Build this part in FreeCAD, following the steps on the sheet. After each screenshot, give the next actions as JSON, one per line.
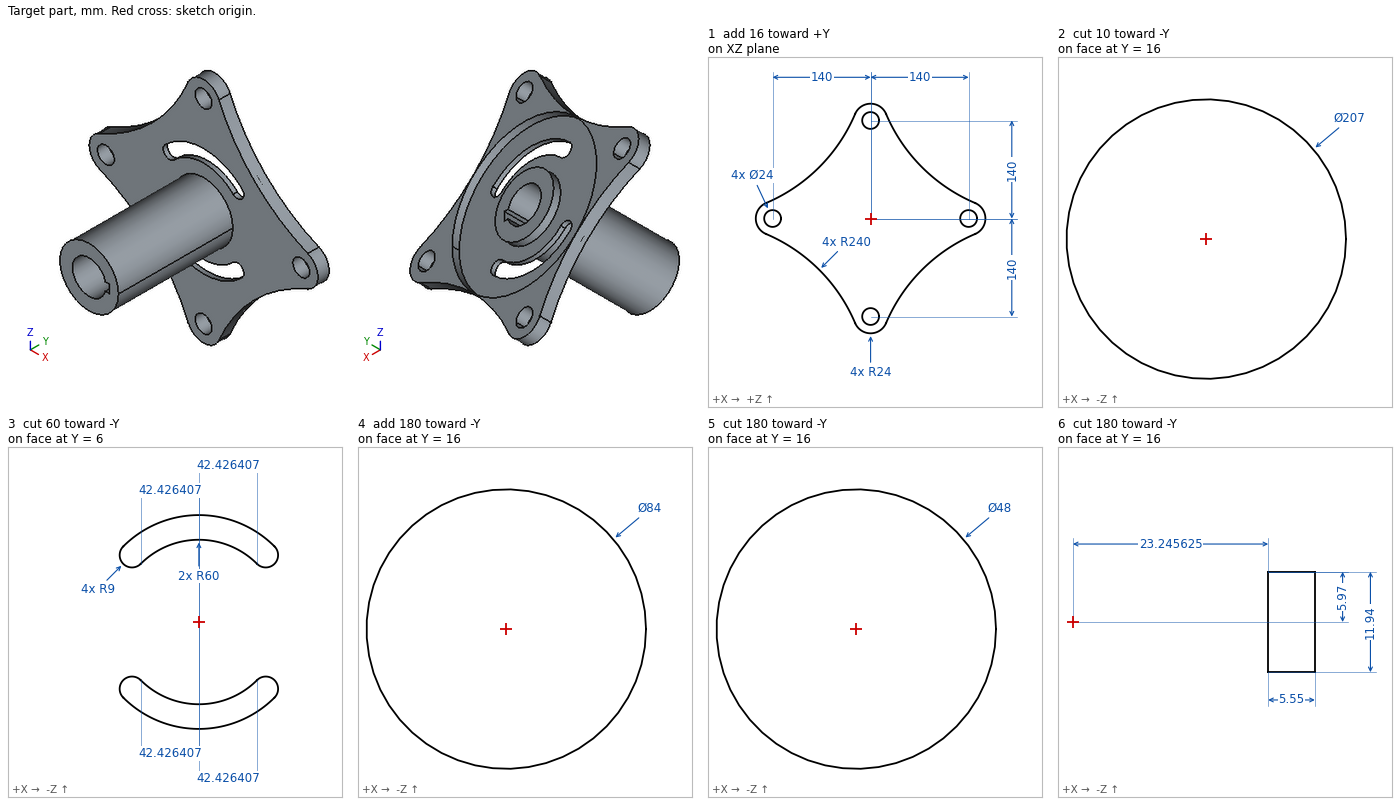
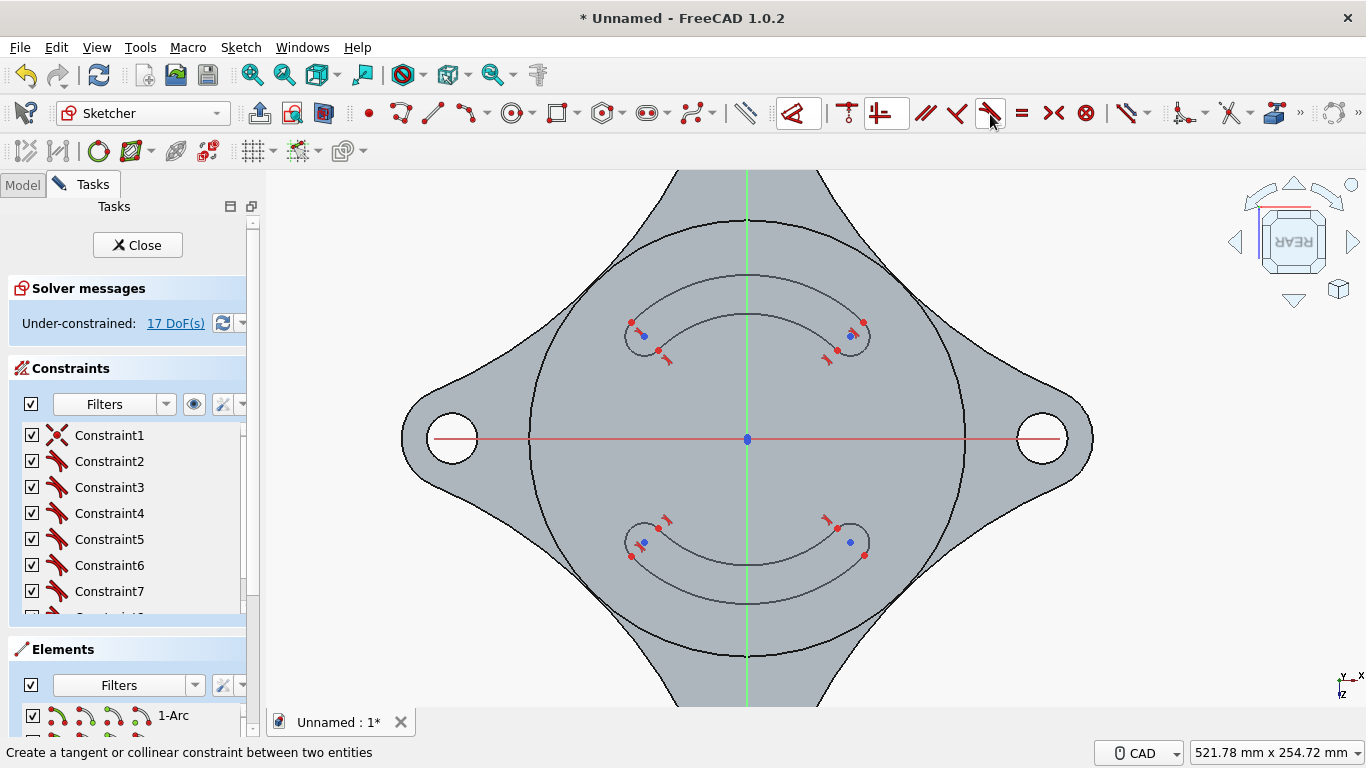
{"action": "left_click", "coordinate": [697, 596]}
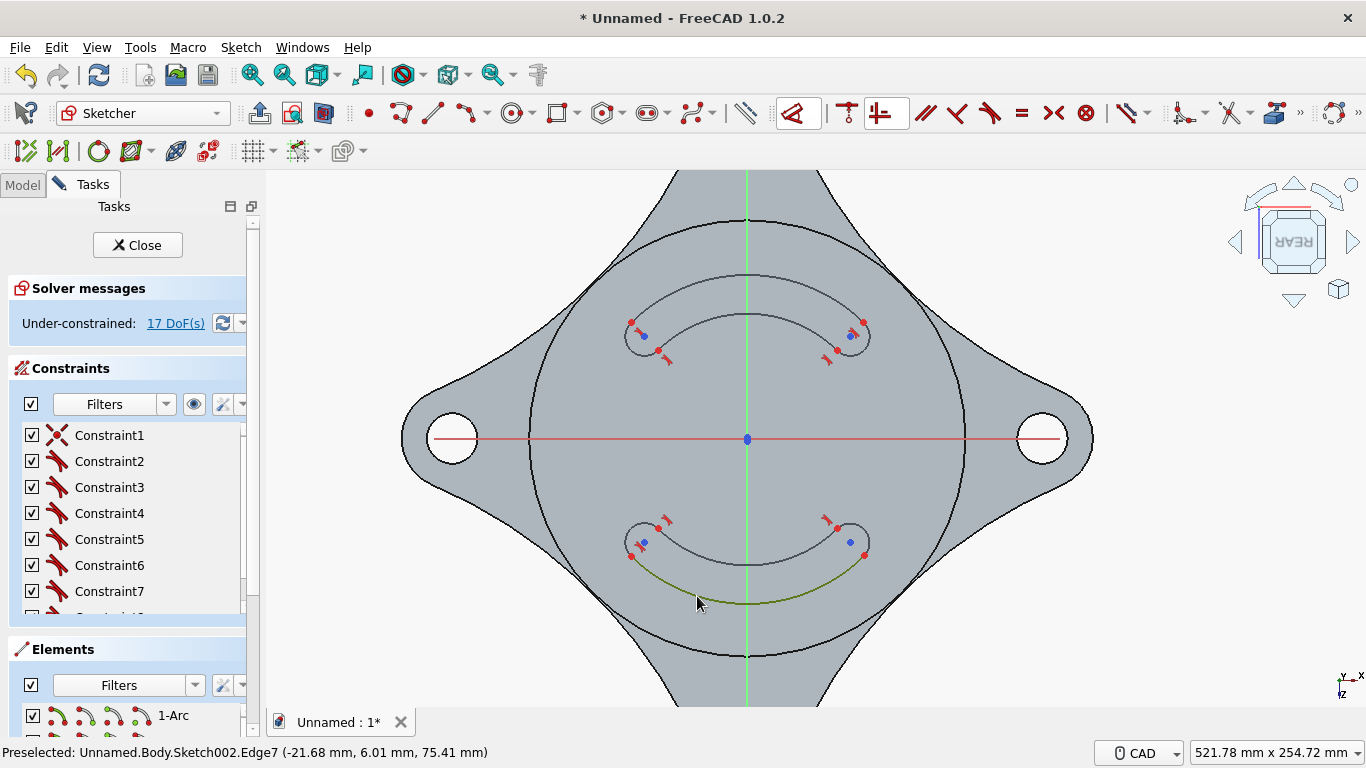
{"action": "left_click", "coordinate": [869, 540]}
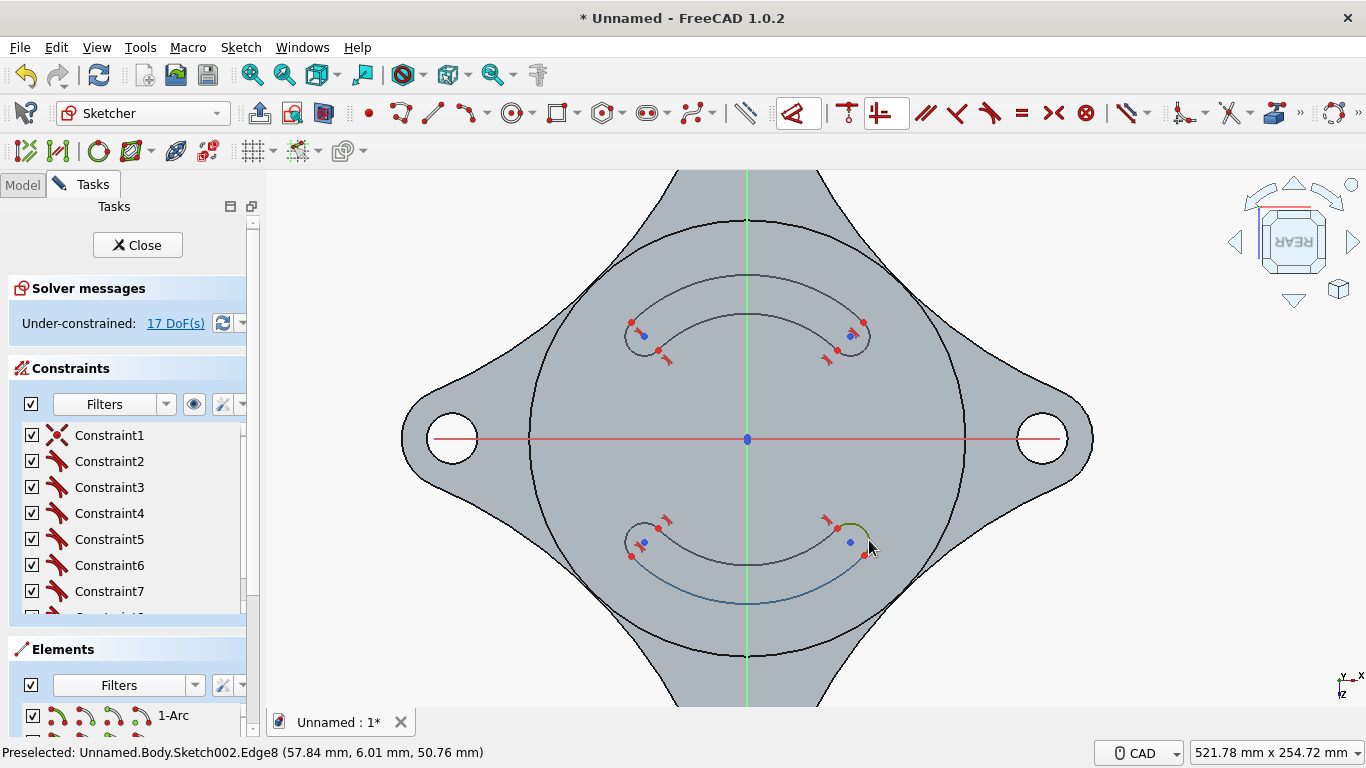
{"action": "left_click", "coordinate": [990, 114]}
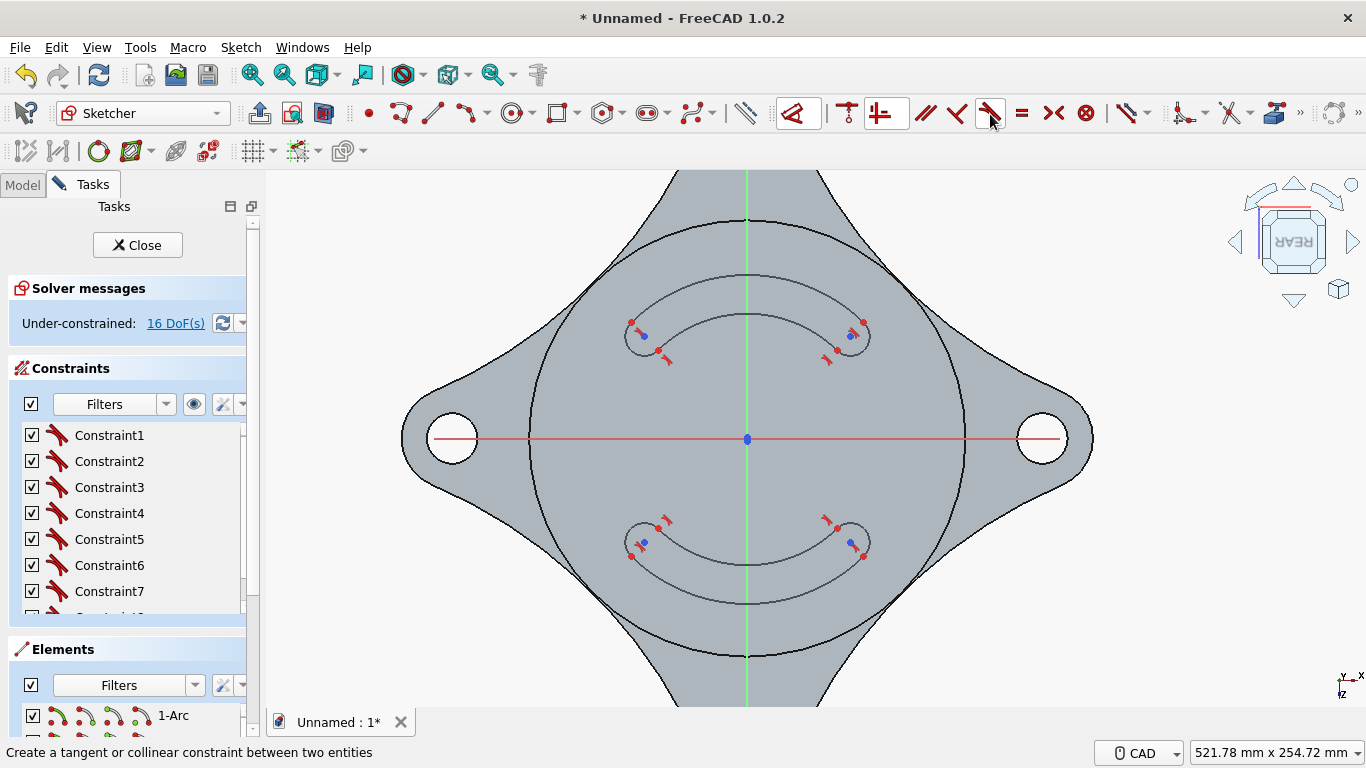
{"action": "left_click", "coordinate": [787, 320]}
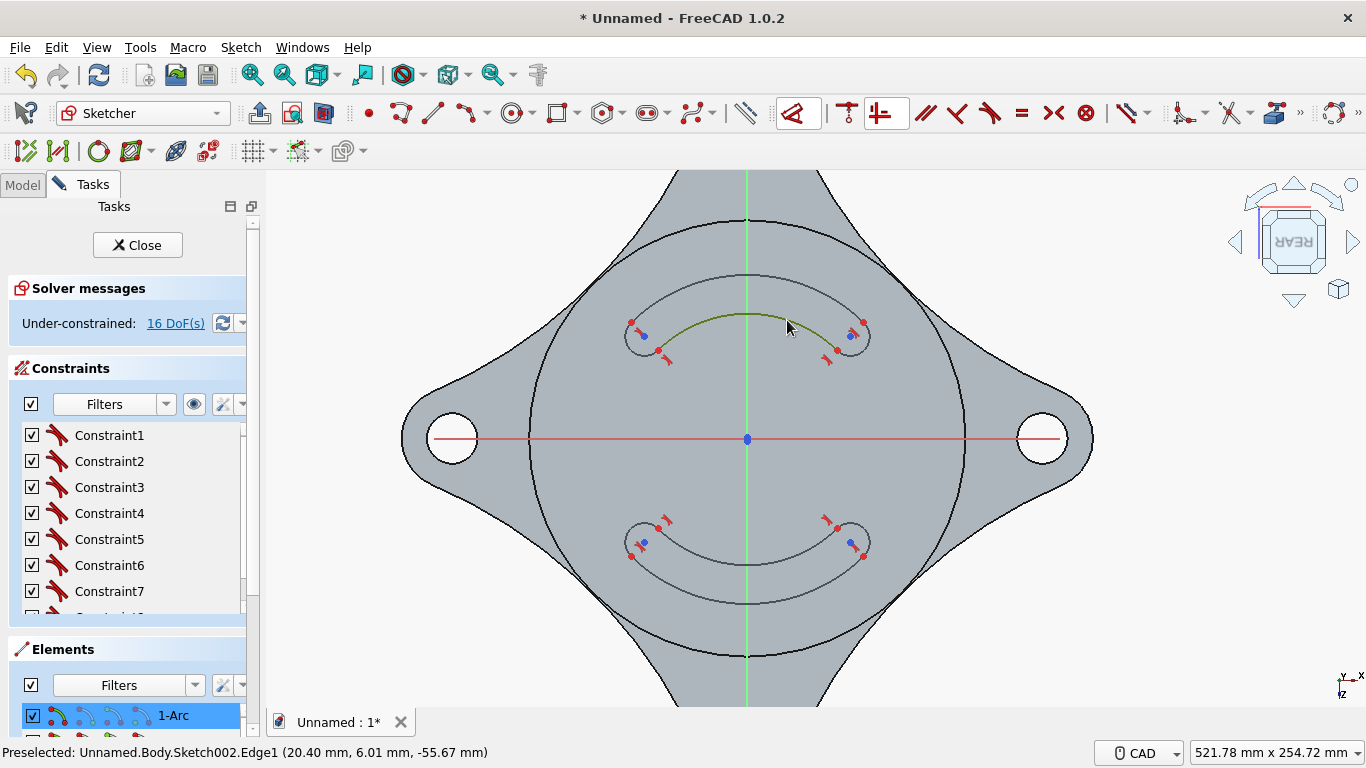
{"action": "left_click", "coordinate": [798, 283]}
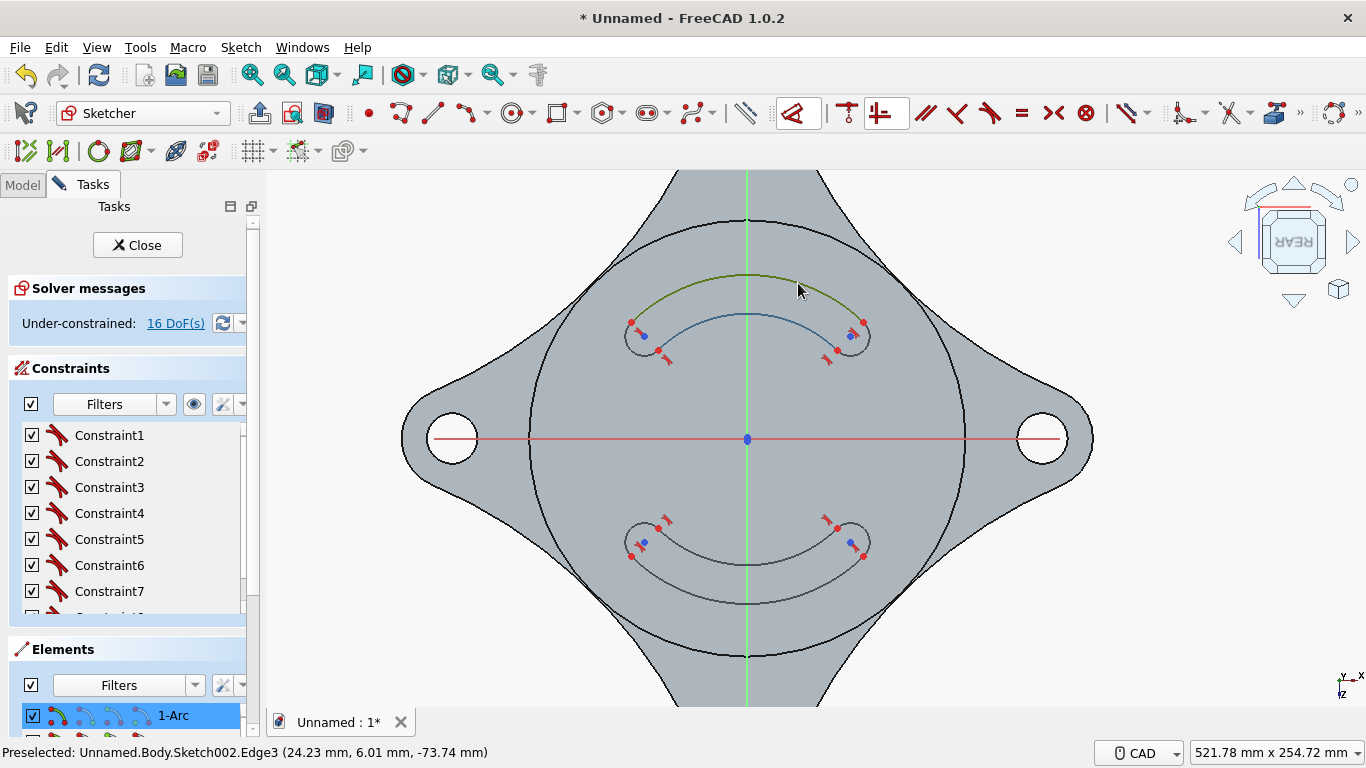
{"action": "left_click", "coordinate": [848, 114]}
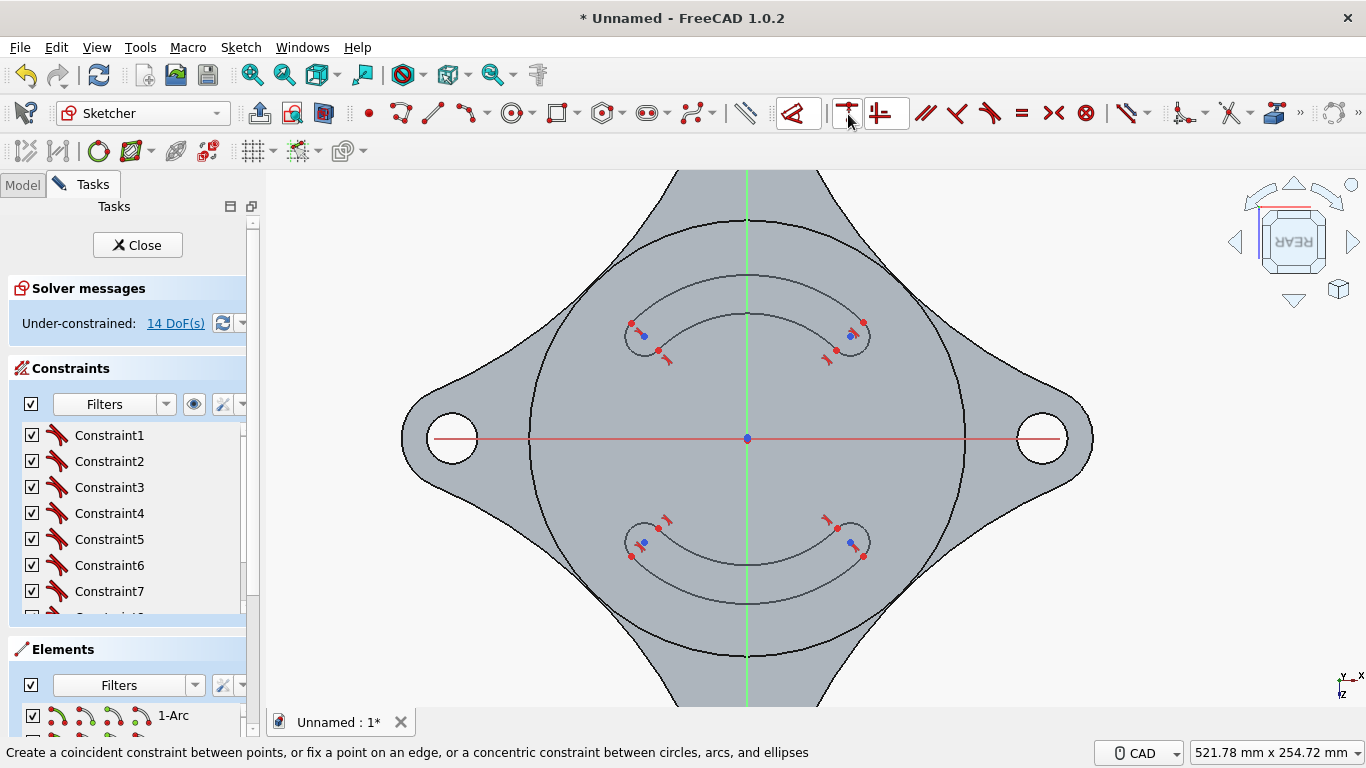
{"action": "left_click", "coordinate": [787, 320]}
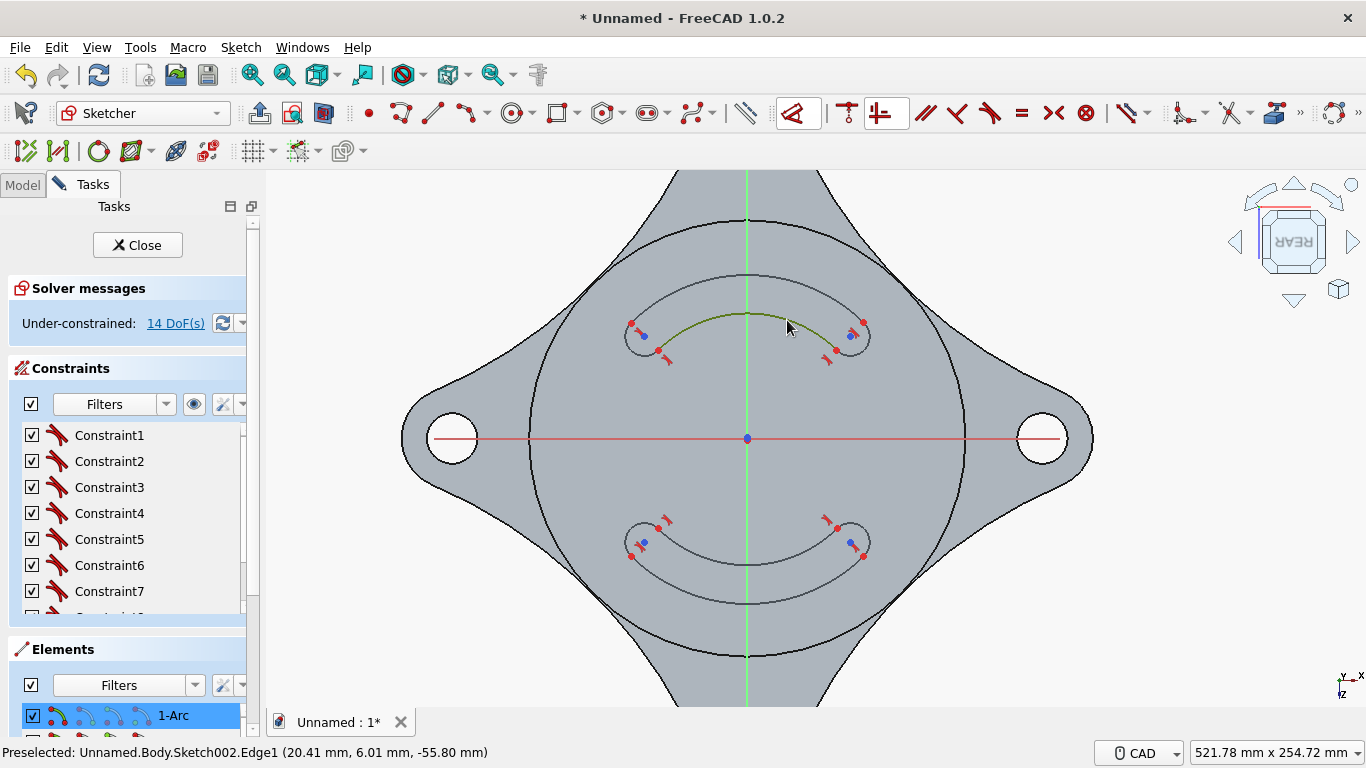
{"action": "left_click", "coordinate": [708, 559]}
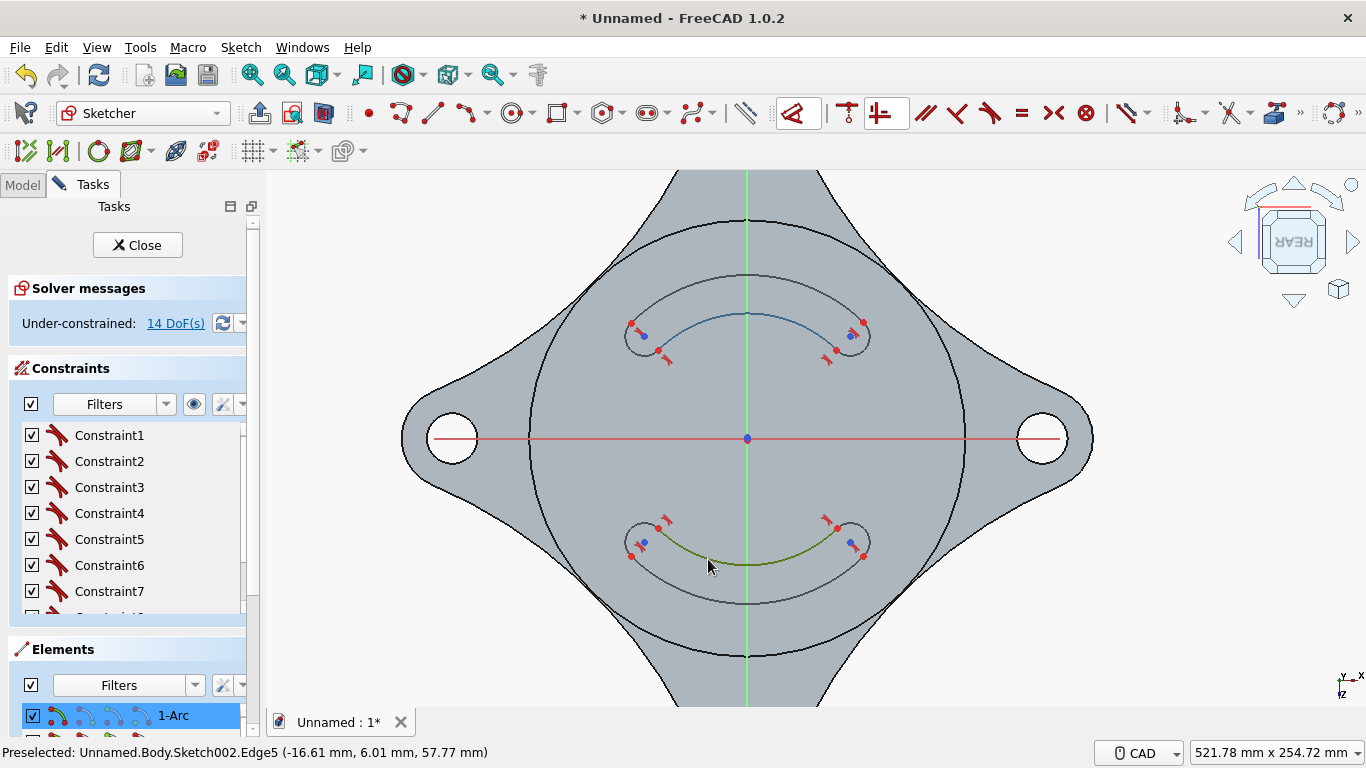
{"action": "left_click", "coordinate": [848, 114]}